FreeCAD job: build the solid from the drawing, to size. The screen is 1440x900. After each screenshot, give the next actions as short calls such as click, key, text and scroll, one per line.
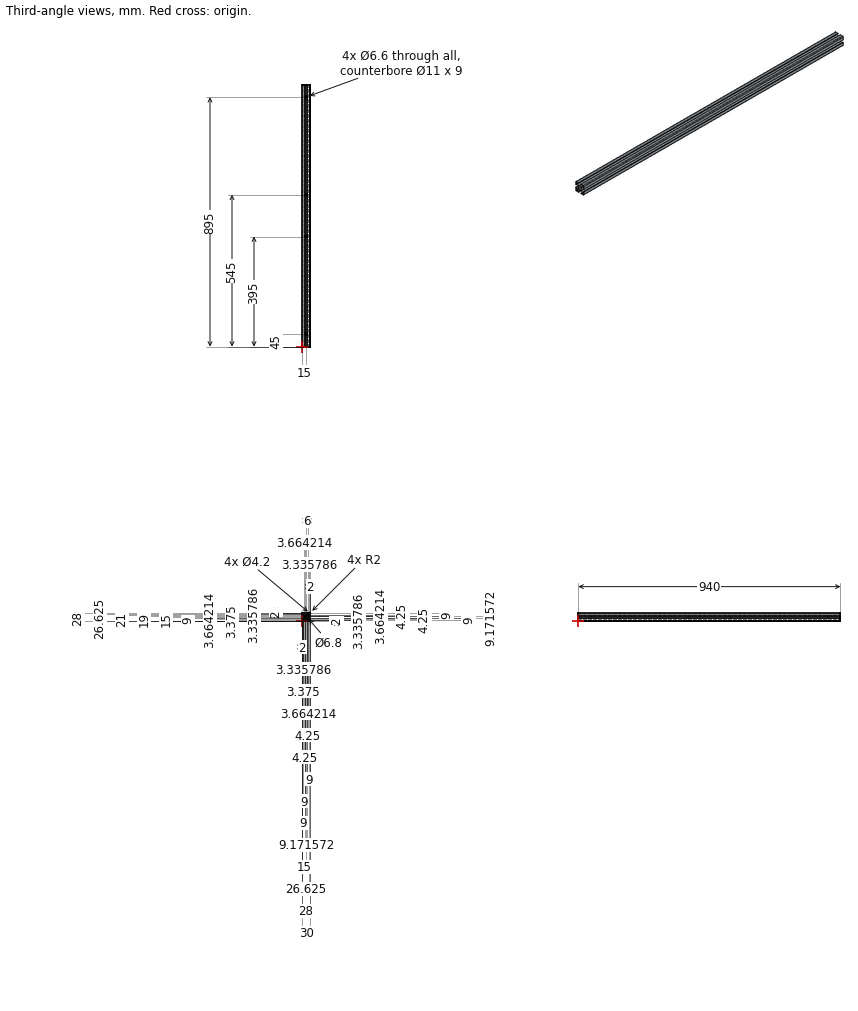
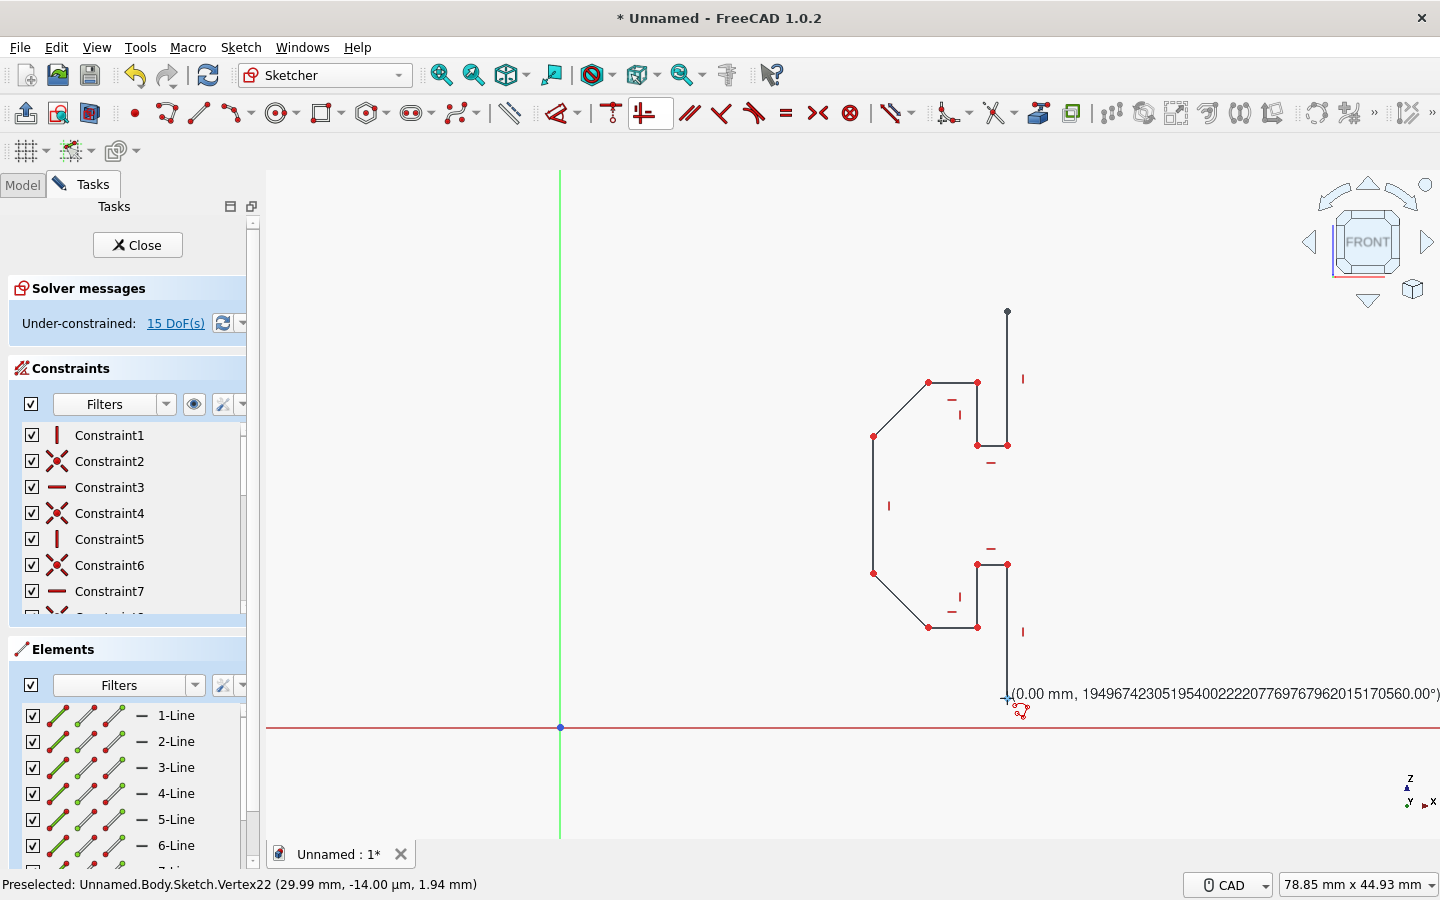
click(977, 728)
click(843, 719)
click(843, 698)
click(907, 698)
click(907, 648)
click(852, 594)
click(716, 594)
click(661, 648)
click(661, 698)
click(724, 698)
click(724, 728)
click(590, 719)
right_click(590, 719)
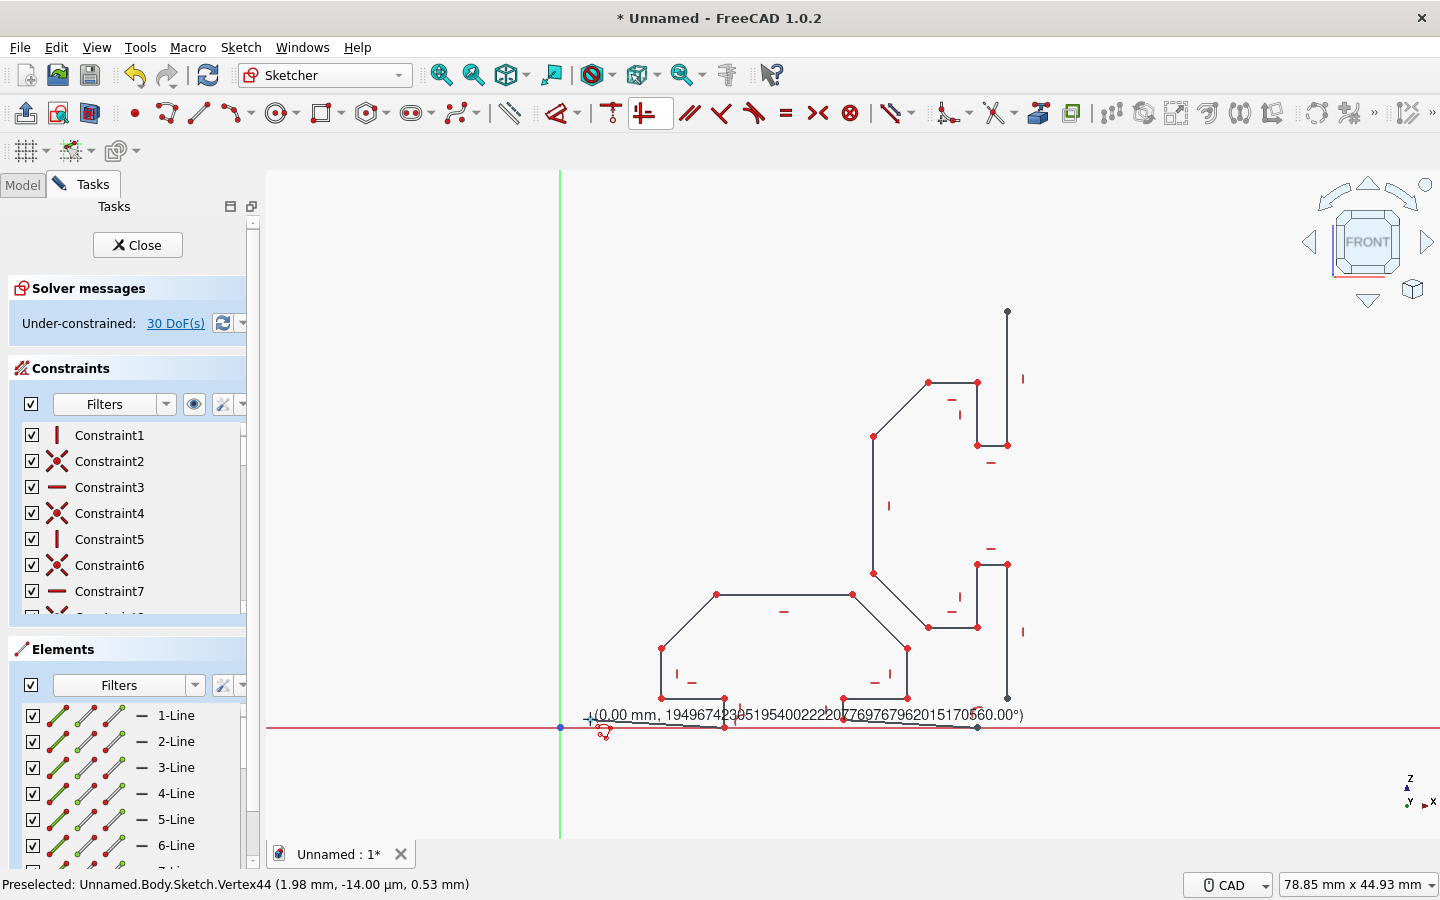
click(560, 698)
click(569, 564)
click(590, 564)
click(590, 627)
click(640, 627)
click(694, 573)
click(694, 436)
click(640, 382)
click(590, 382)
click(590, 445)
click(560, 445)
click(569, 311)
right_click(569, 311)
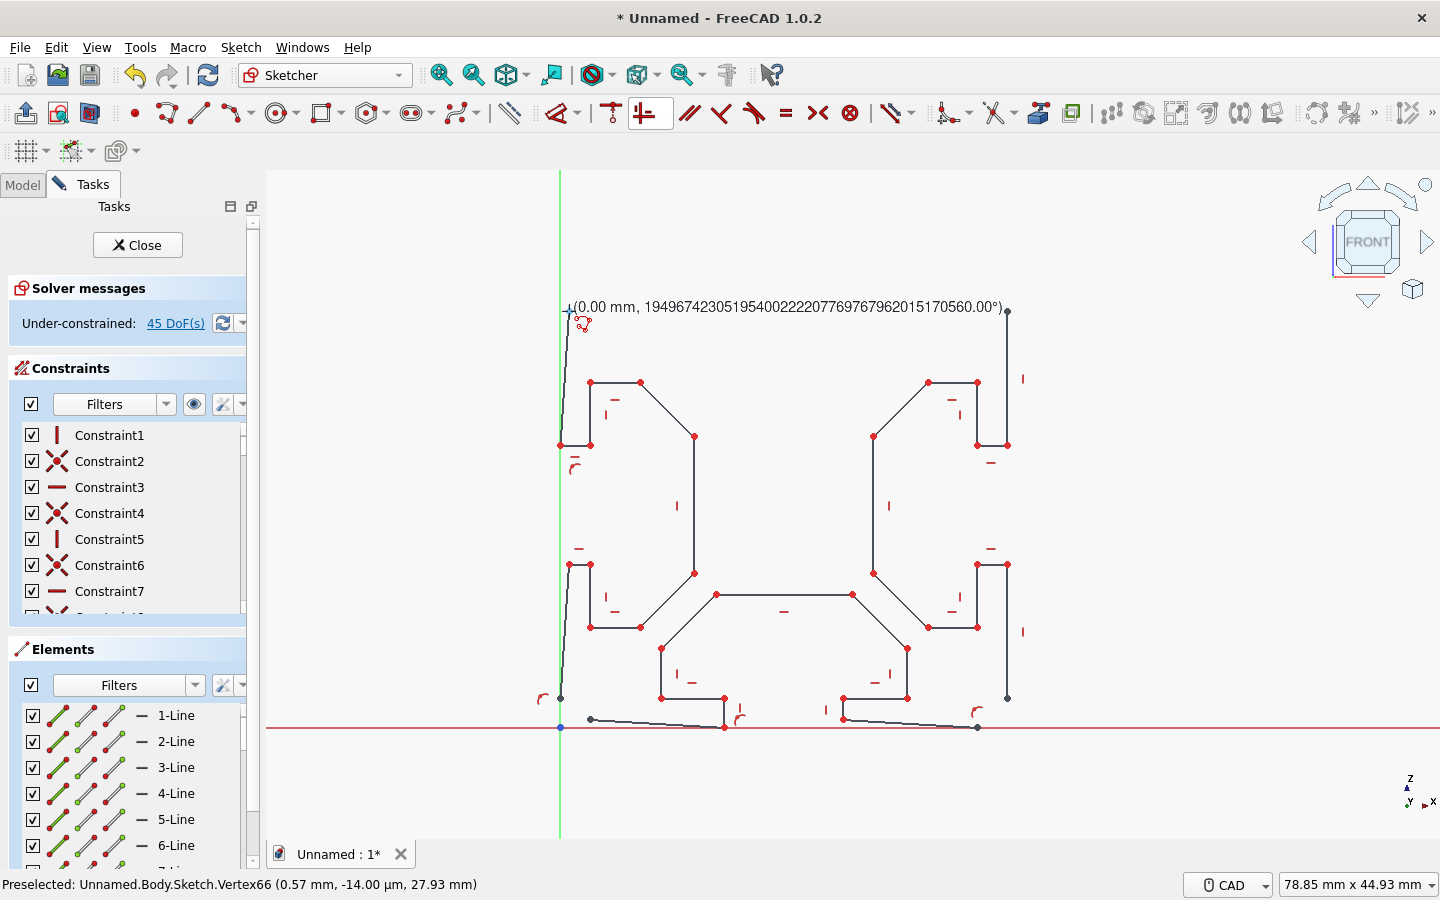
click(590, 281)
click(724, 281)
click(724, 311)
click(661, 311)
click(661, 361)
click(716, 415)
click(852, 415)
click(907, 361)
click(907, 311)
click(843, 311)
click(843, 281)
click(977, 281)
right_click(977, 281)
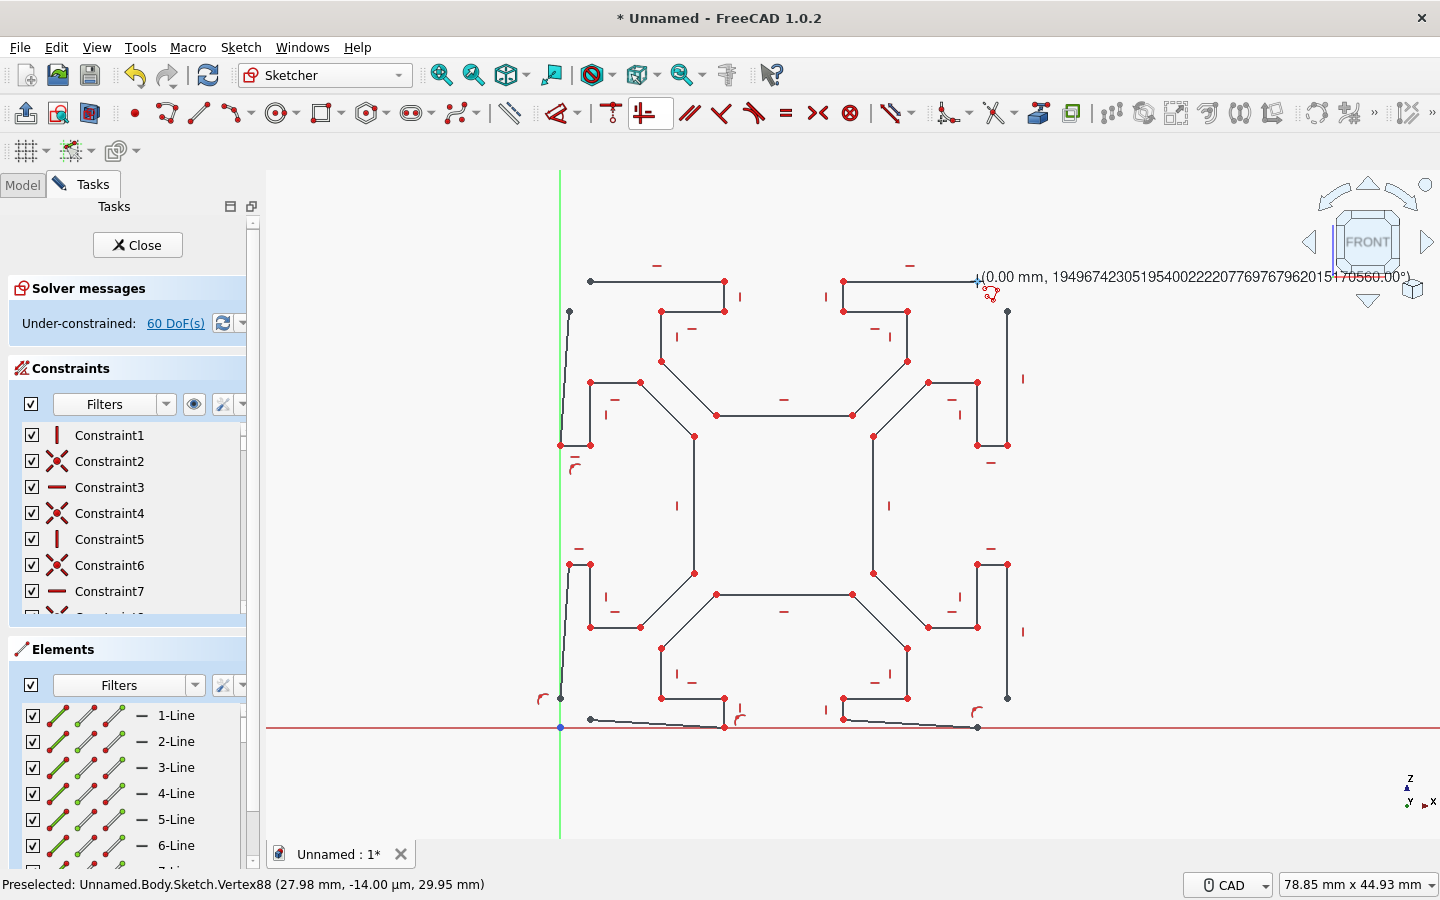
click(232, 114)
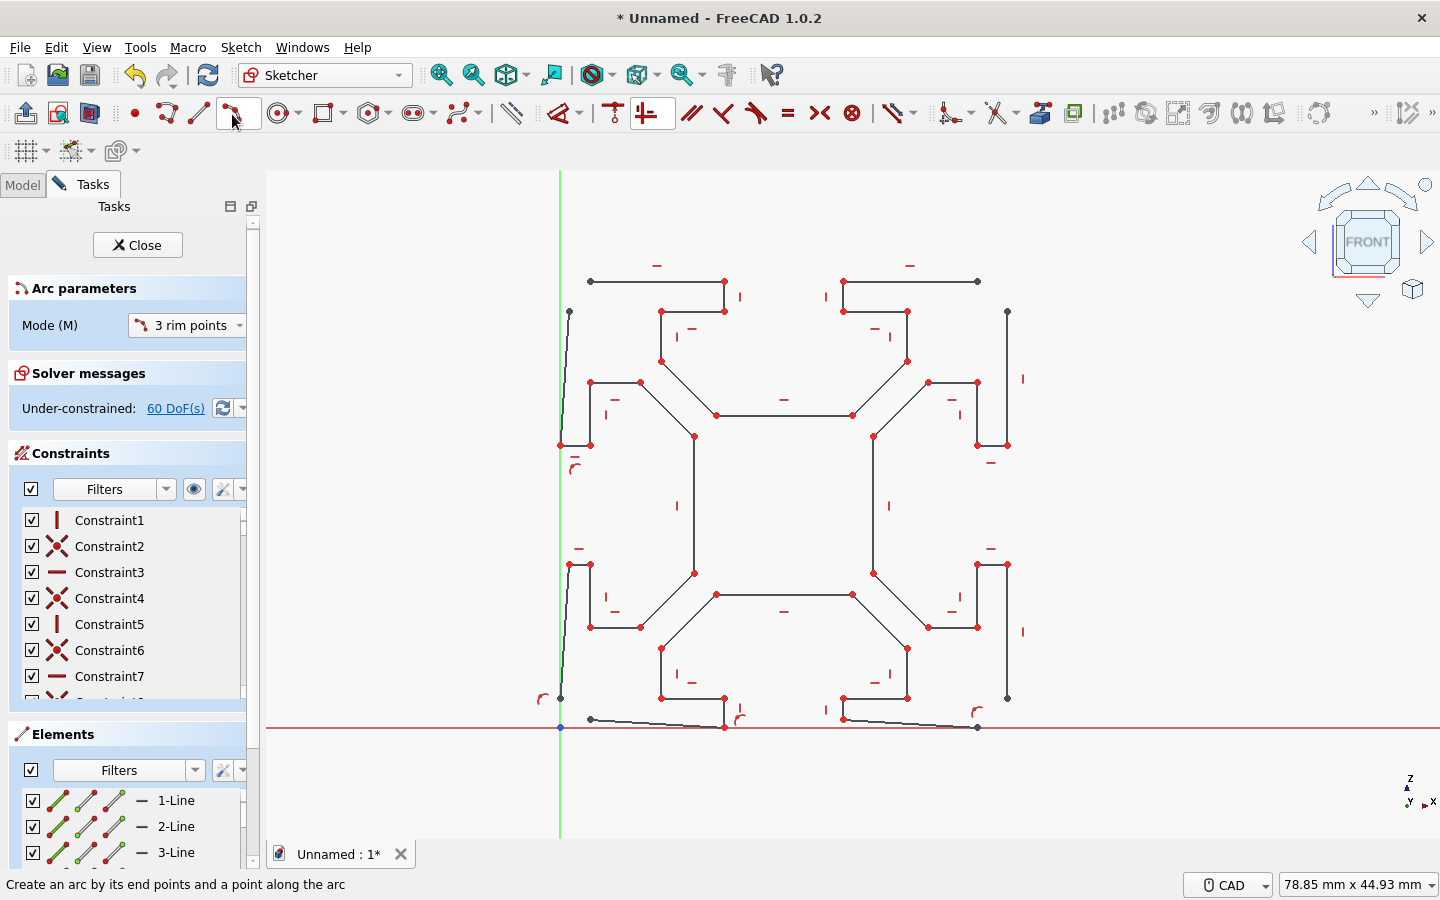
click(1007, 699)
click(977, 728)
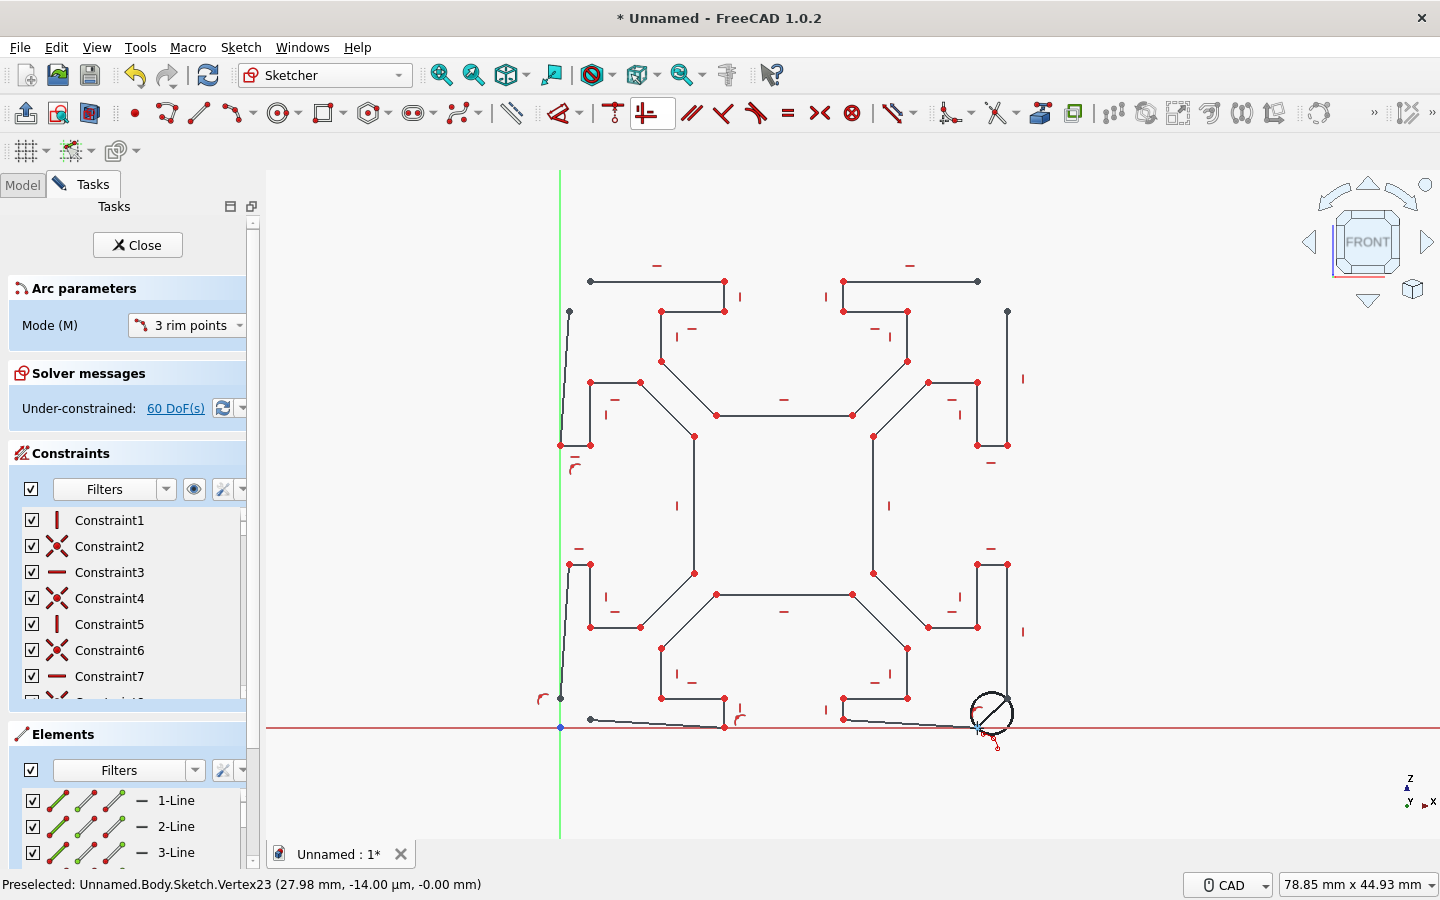
scroll(998, 719, up, 3)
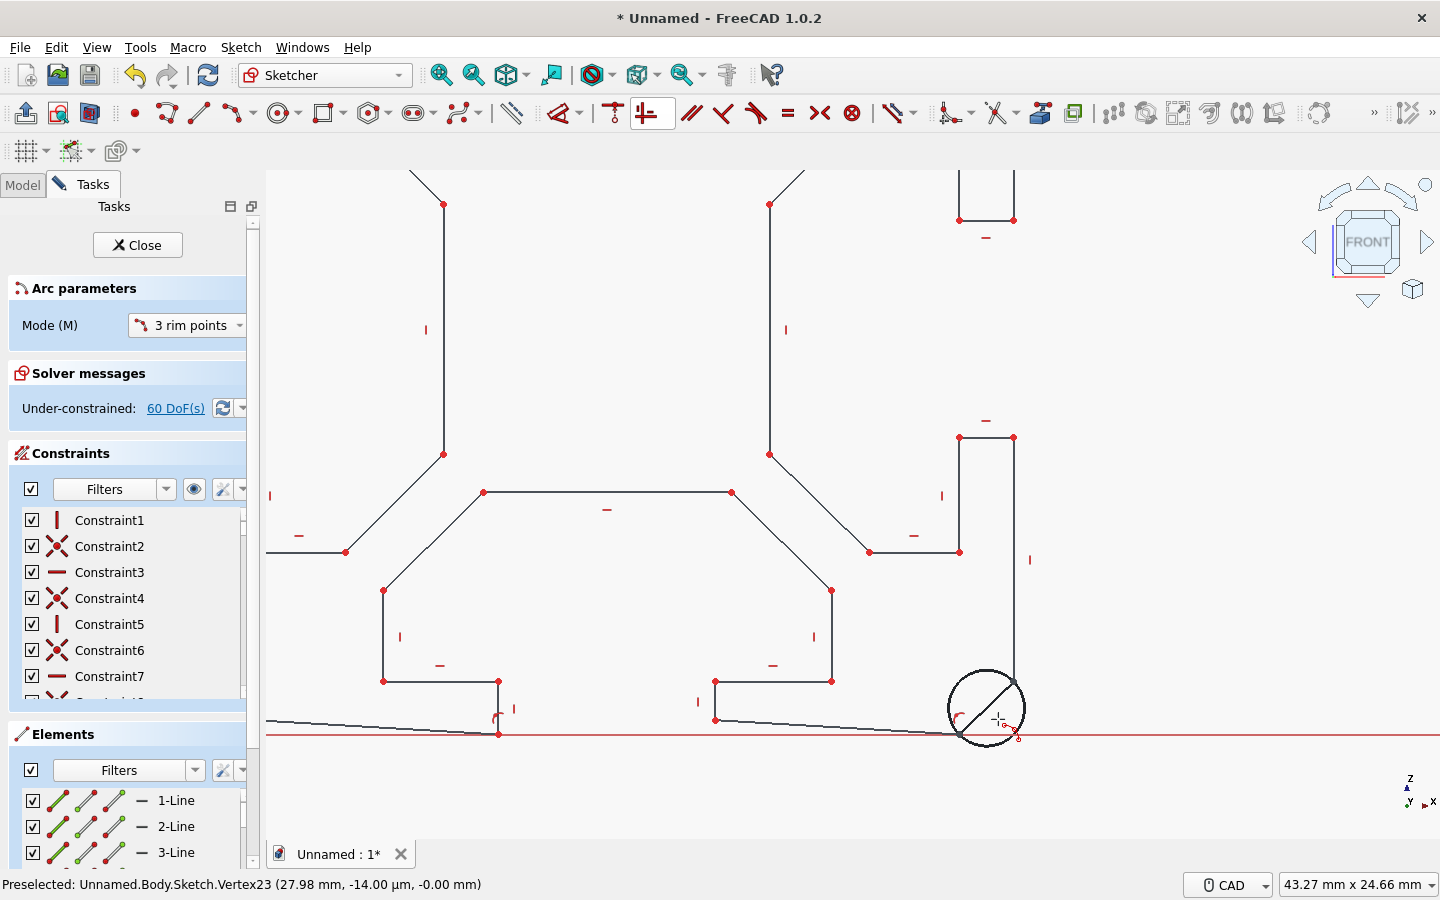
click(998, 719)